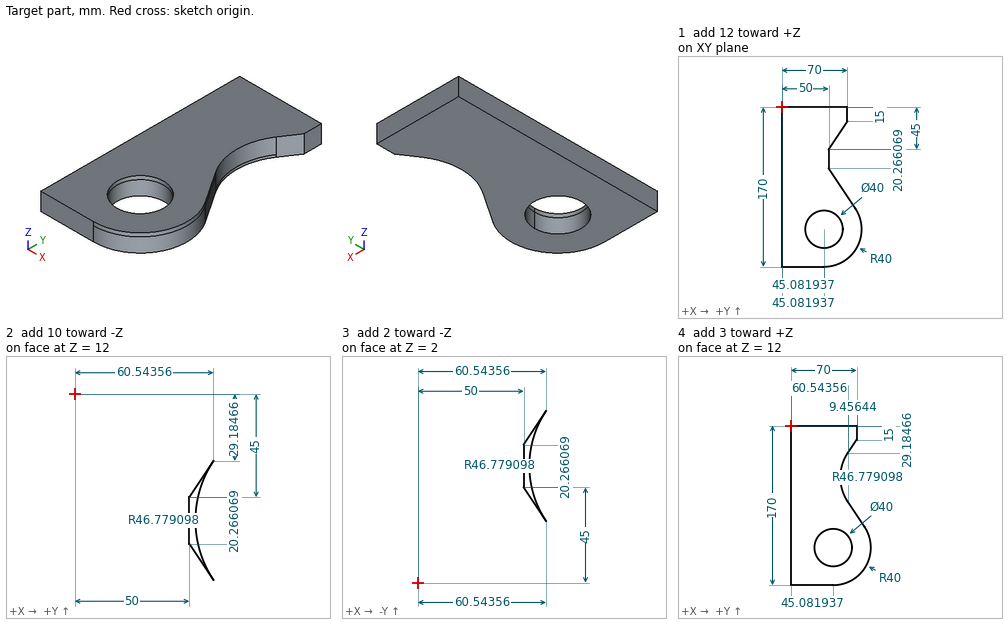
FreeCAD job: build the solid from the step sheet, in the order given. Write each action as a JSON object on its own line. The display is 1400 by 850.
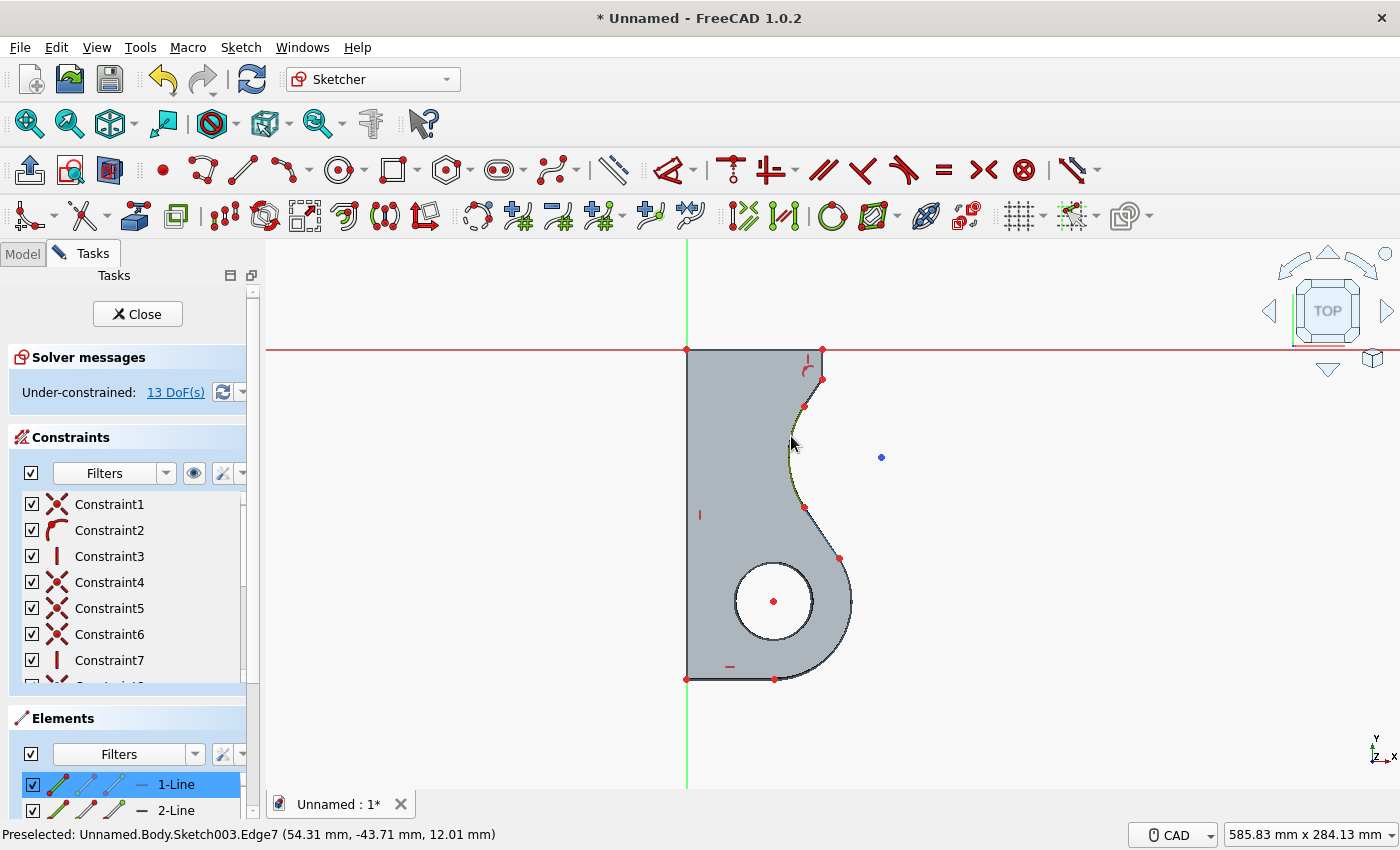
{"action": "left_click", "coordinate": [904, 170]}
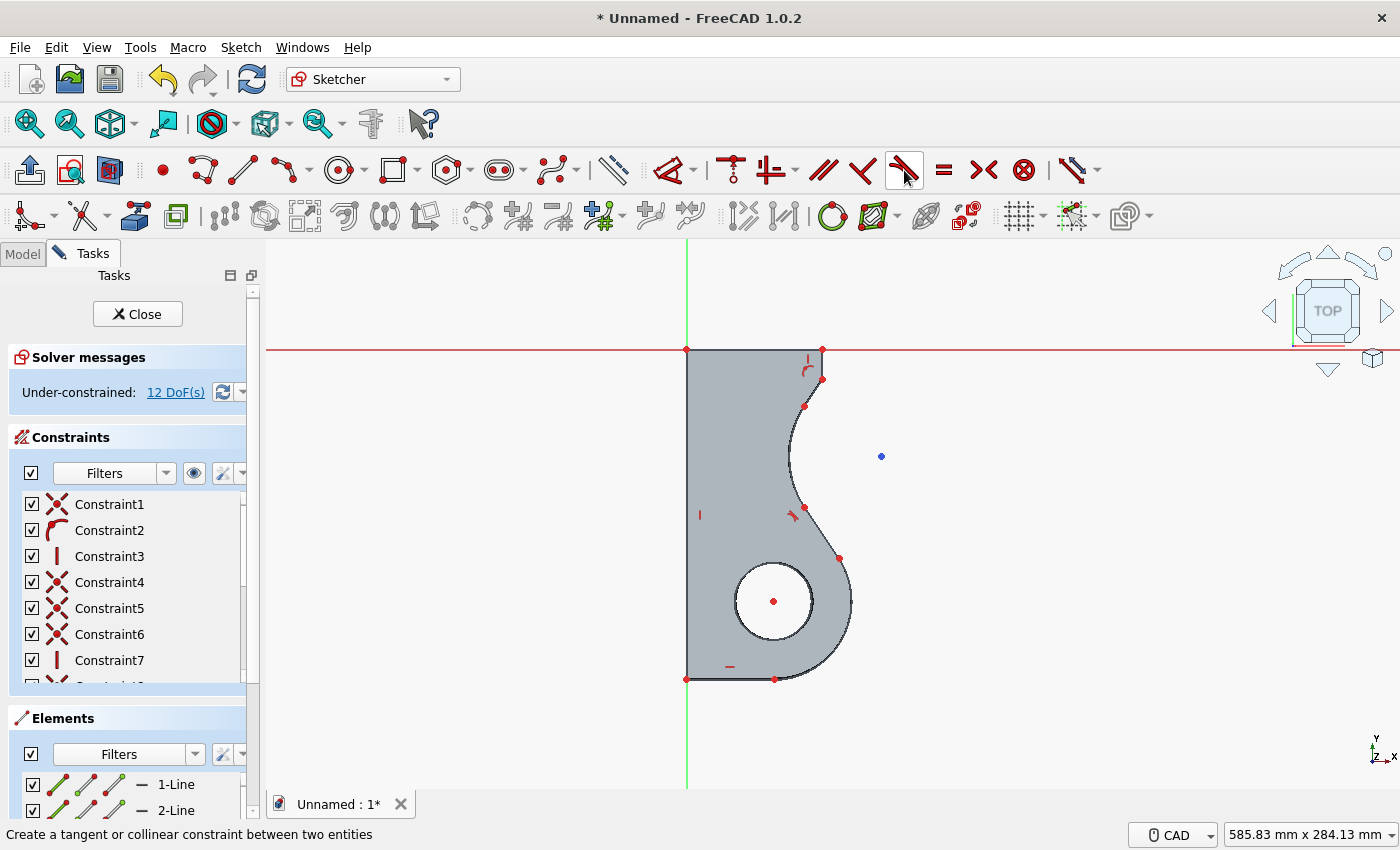
{"action": "left_click", "coordinate": [829, 544]}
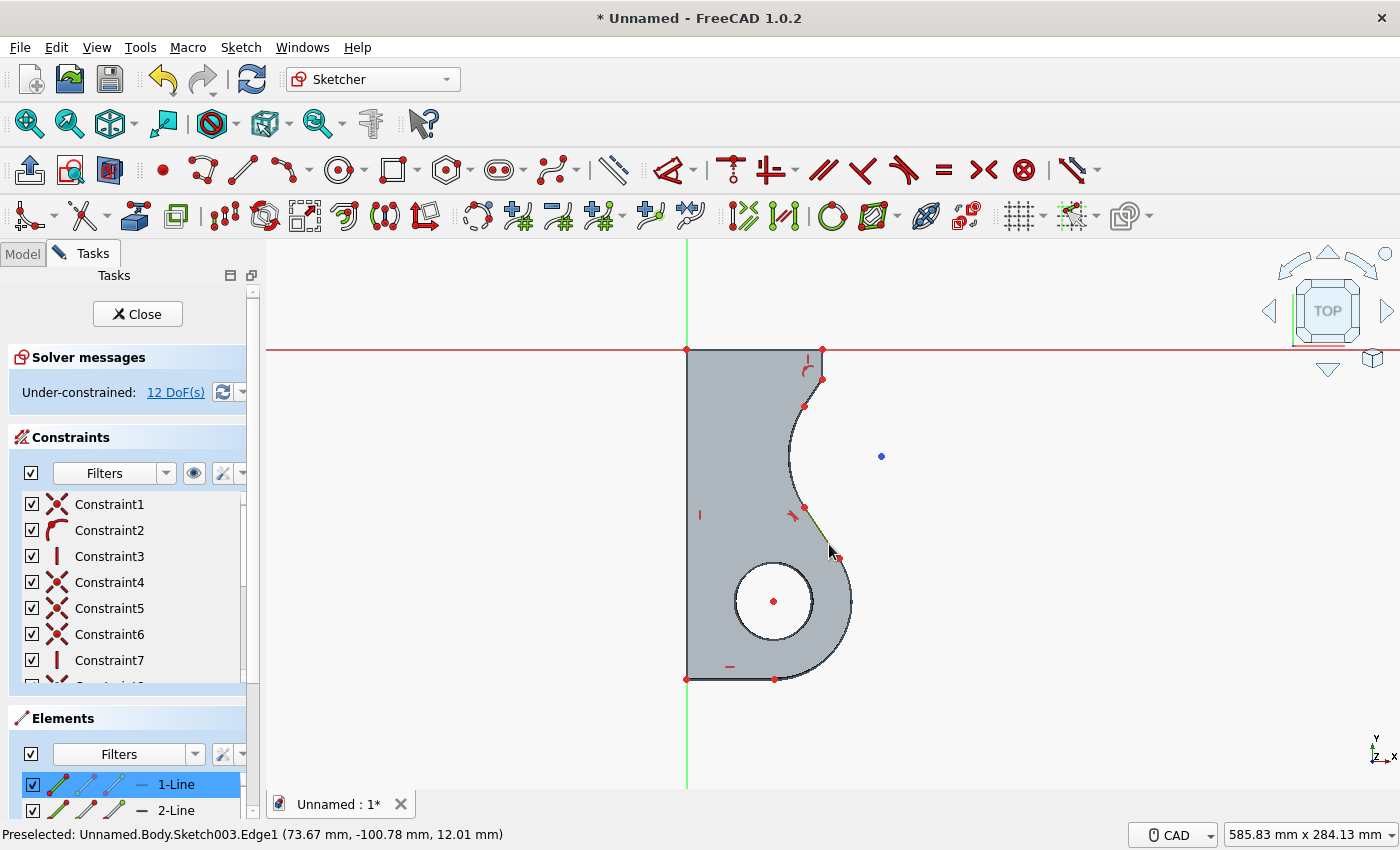
{"action": "left_click", "coordinate": [821, 664]}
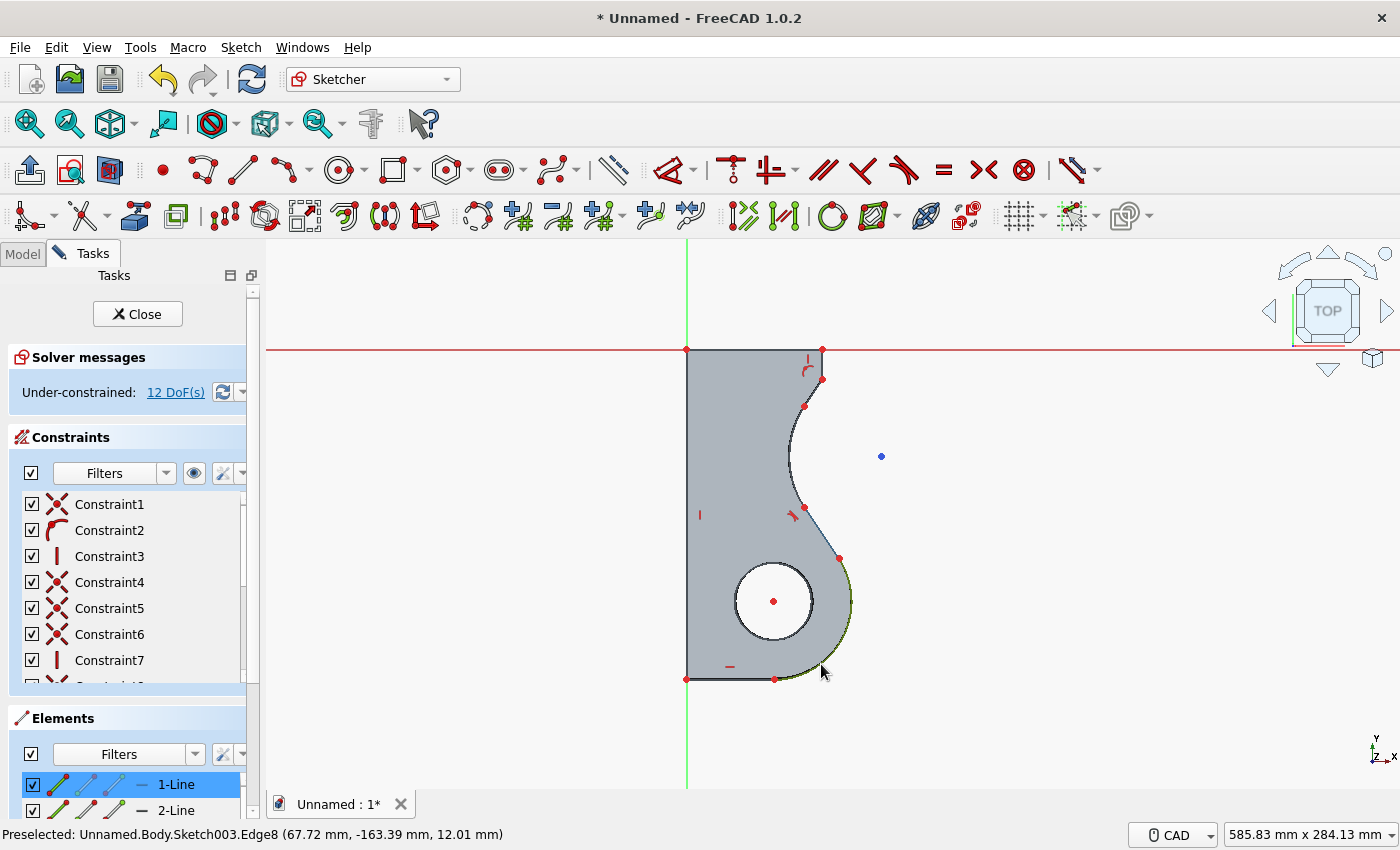
{"action": "left_click", "coordinate": [904, 170]}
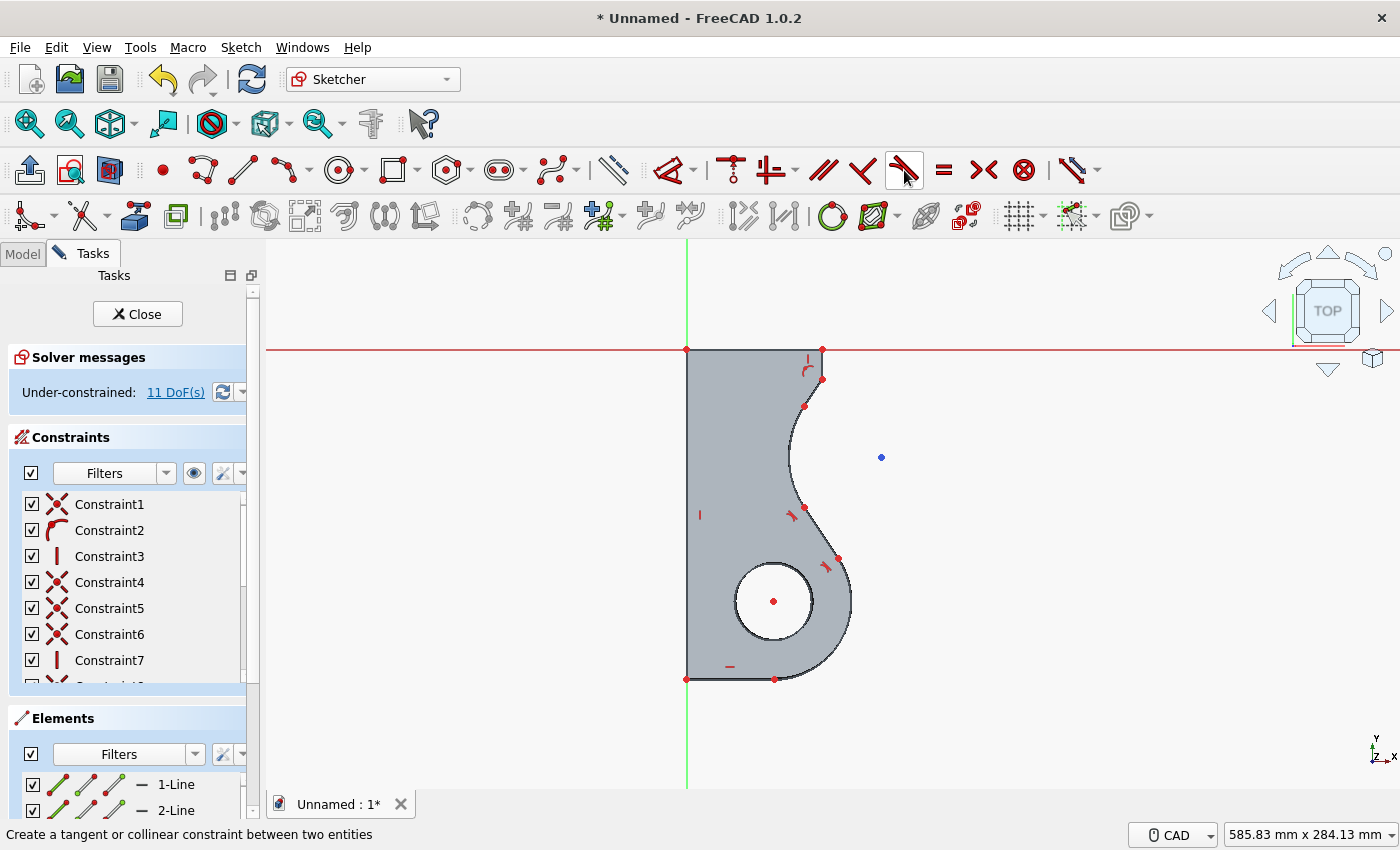
{"action": "scroll", "coordinate": [809, 399], "scroll_direction": "up", "scroll_amount": 2}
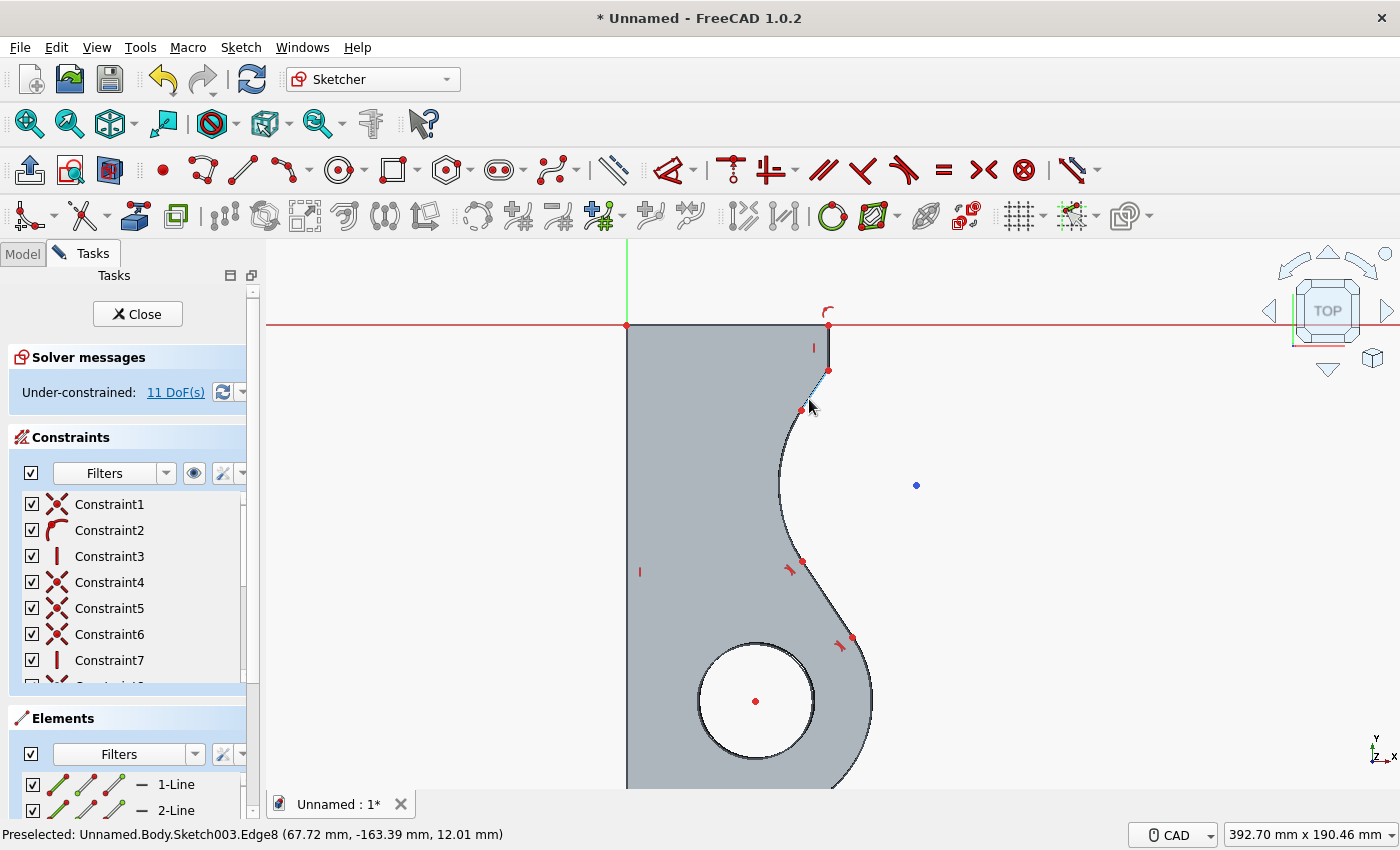
{"action": "left_click", "coordinate": [809, 399]}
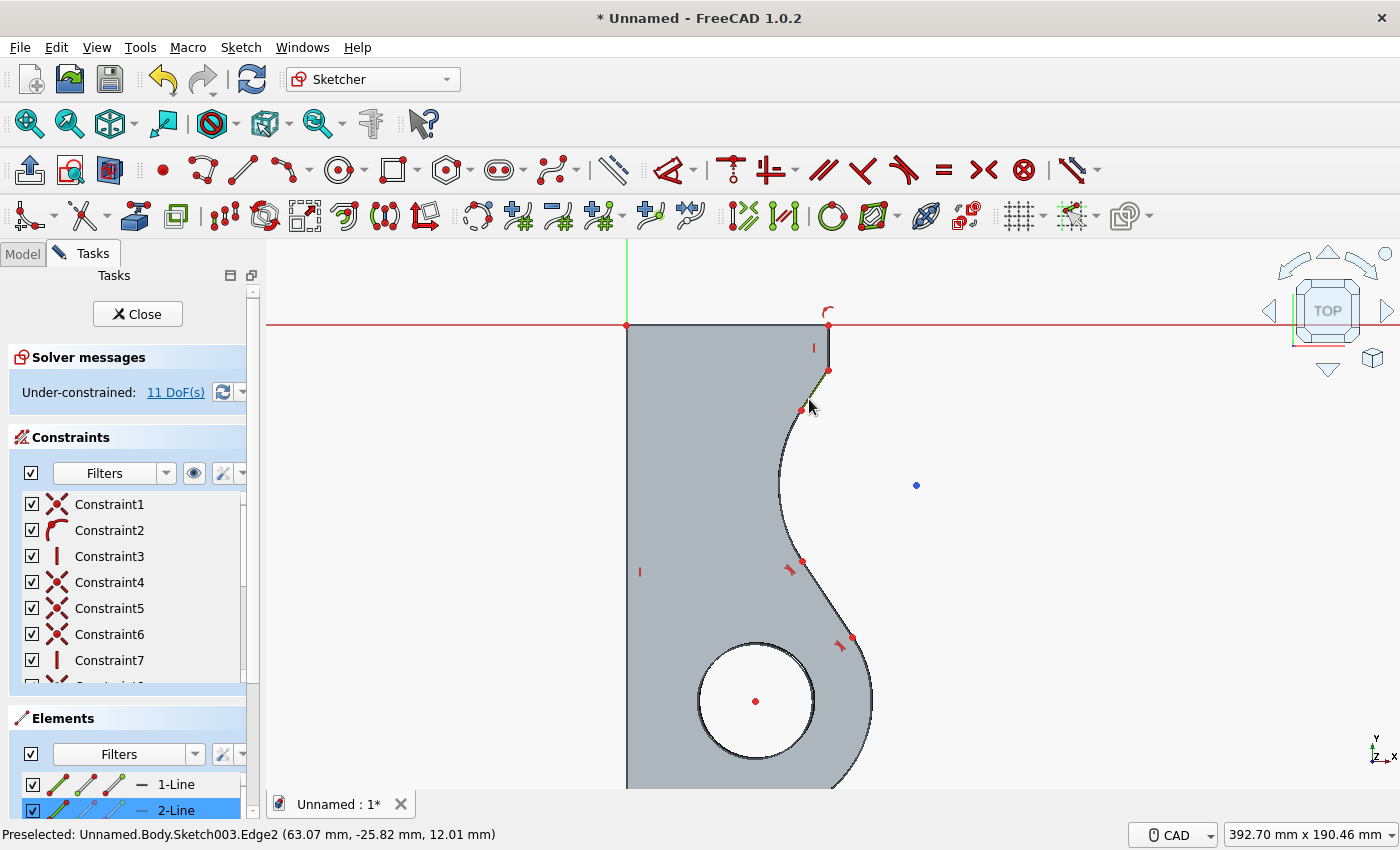
{"action": "left_click", "coordinate": [783, 455]}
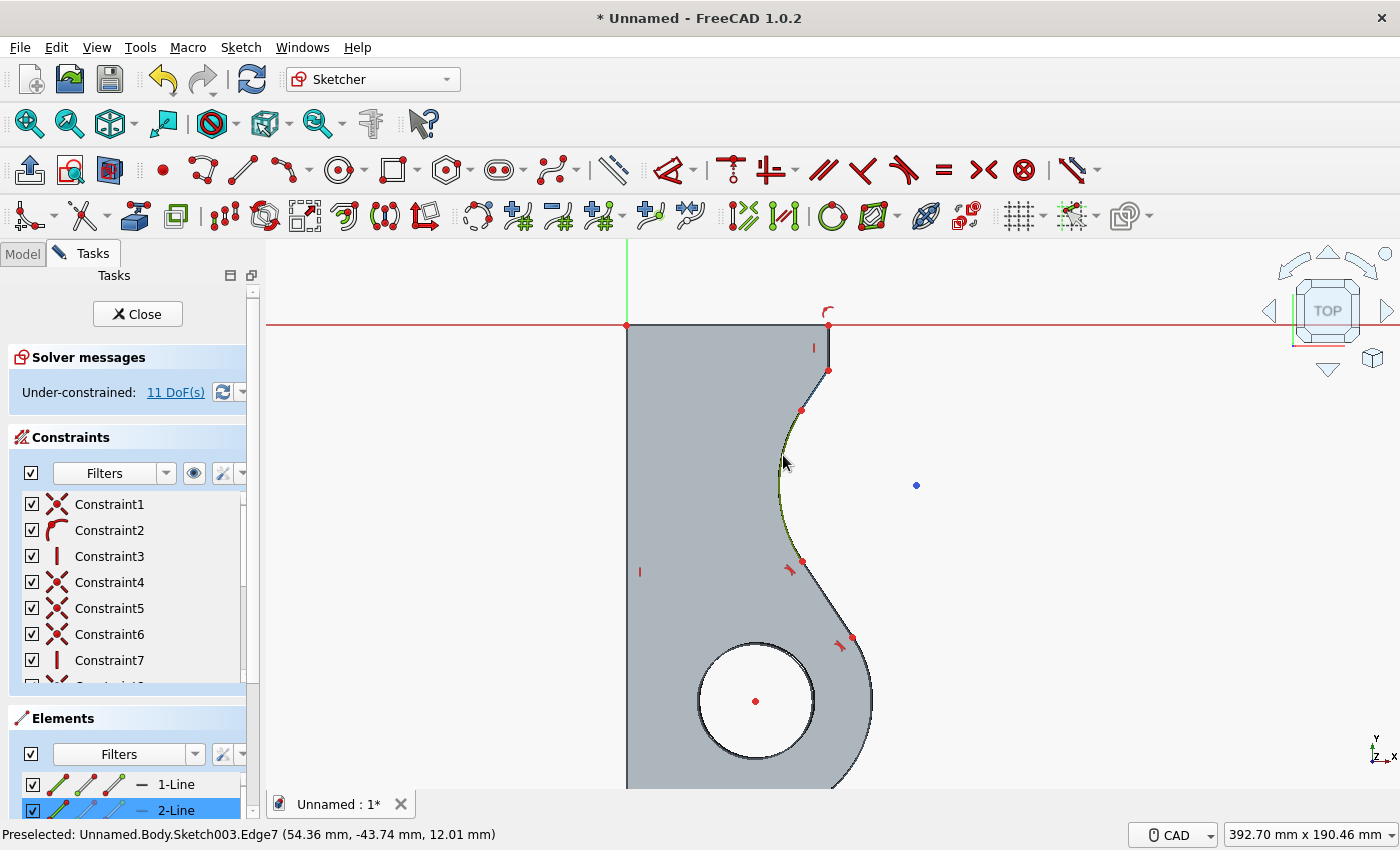
{"action": "left_click", "coordinate": [904, 170]}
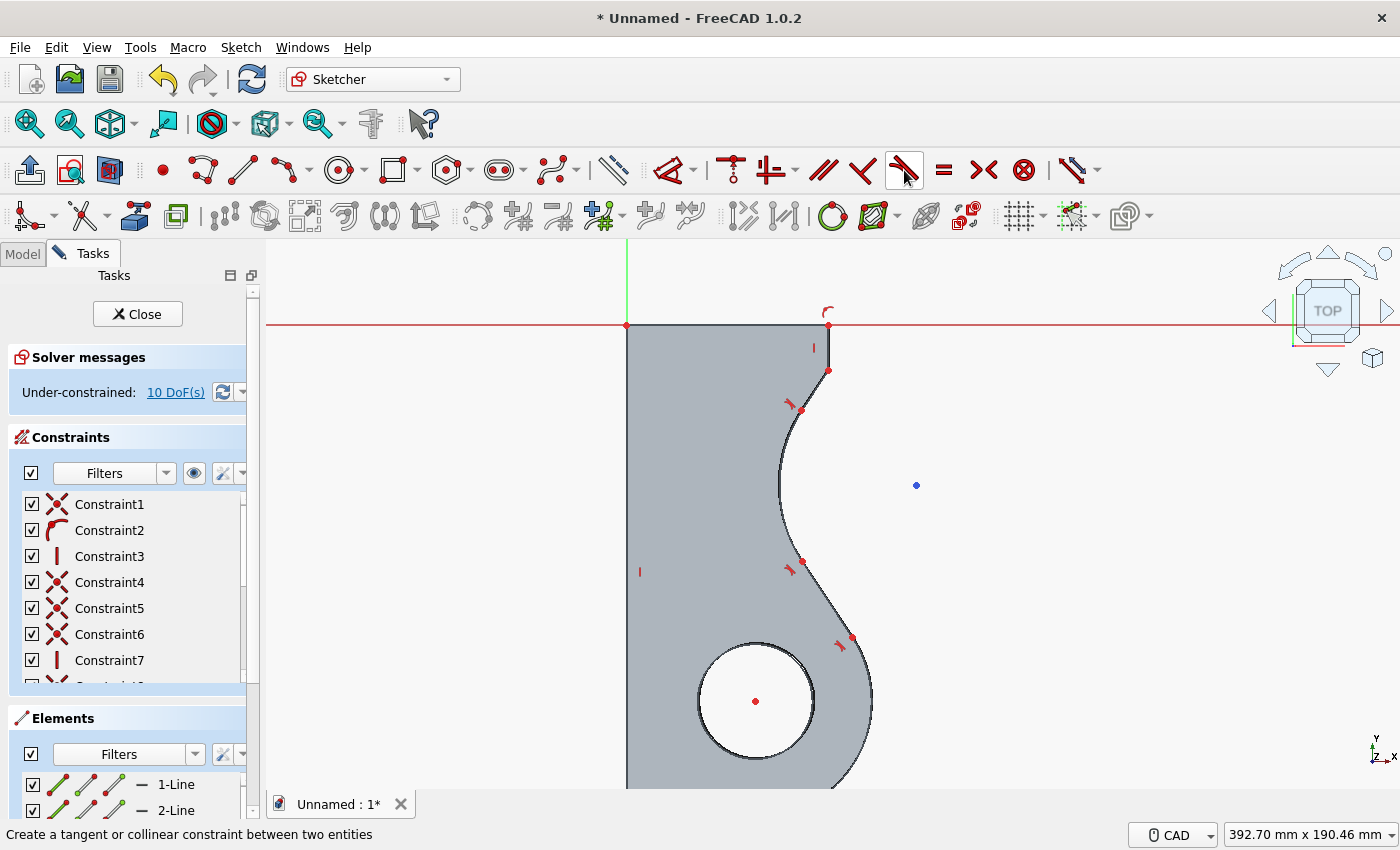
{"action": "left_click", "coordinate": [783, 455]}